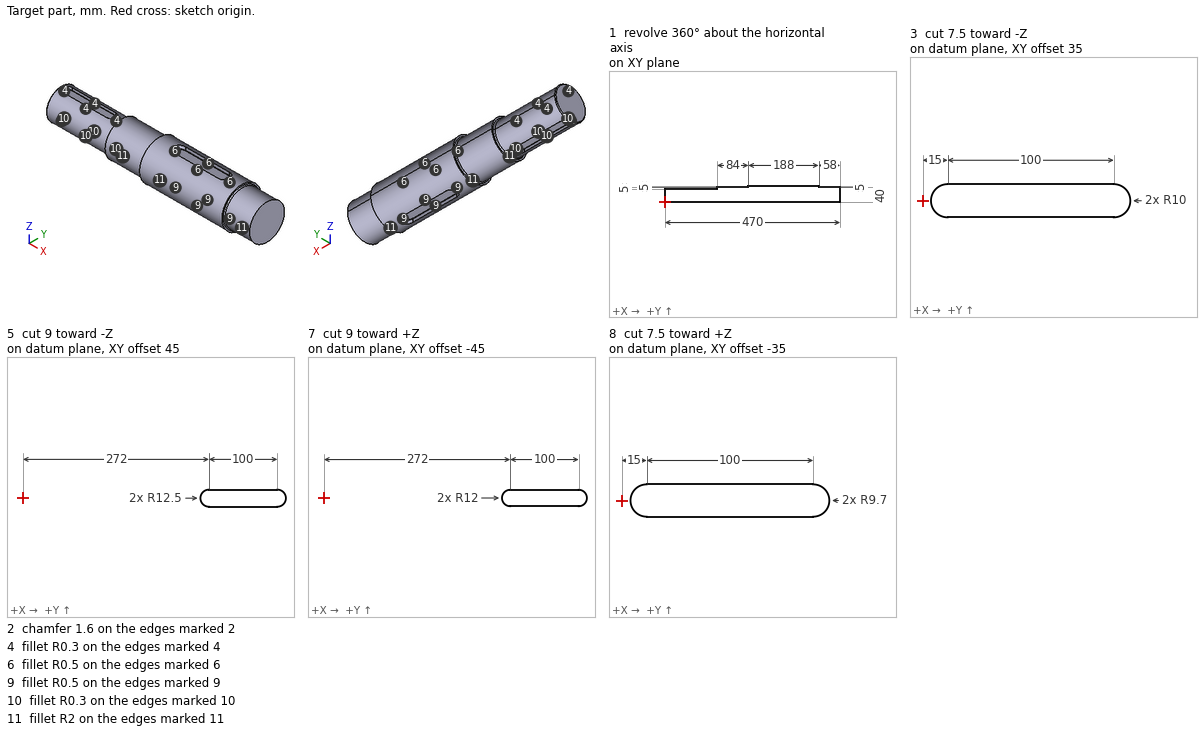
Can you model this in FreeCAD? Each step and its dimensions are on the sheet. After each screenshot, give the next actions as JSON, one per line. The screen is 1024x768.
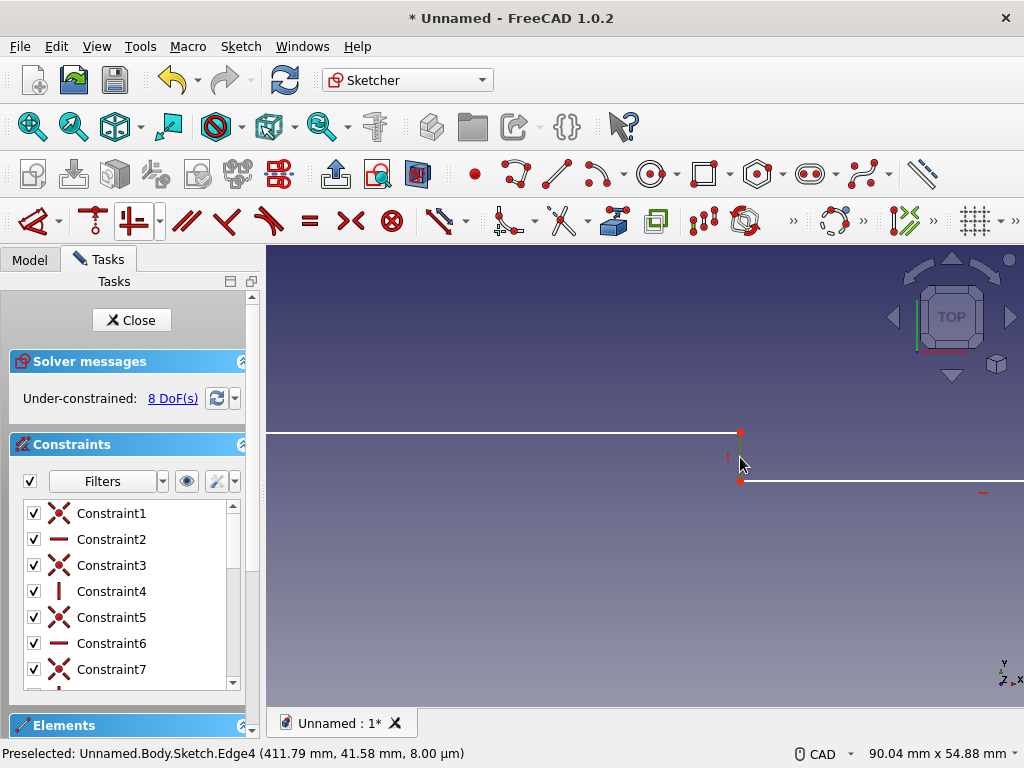
{"action": "key", "text": "i"}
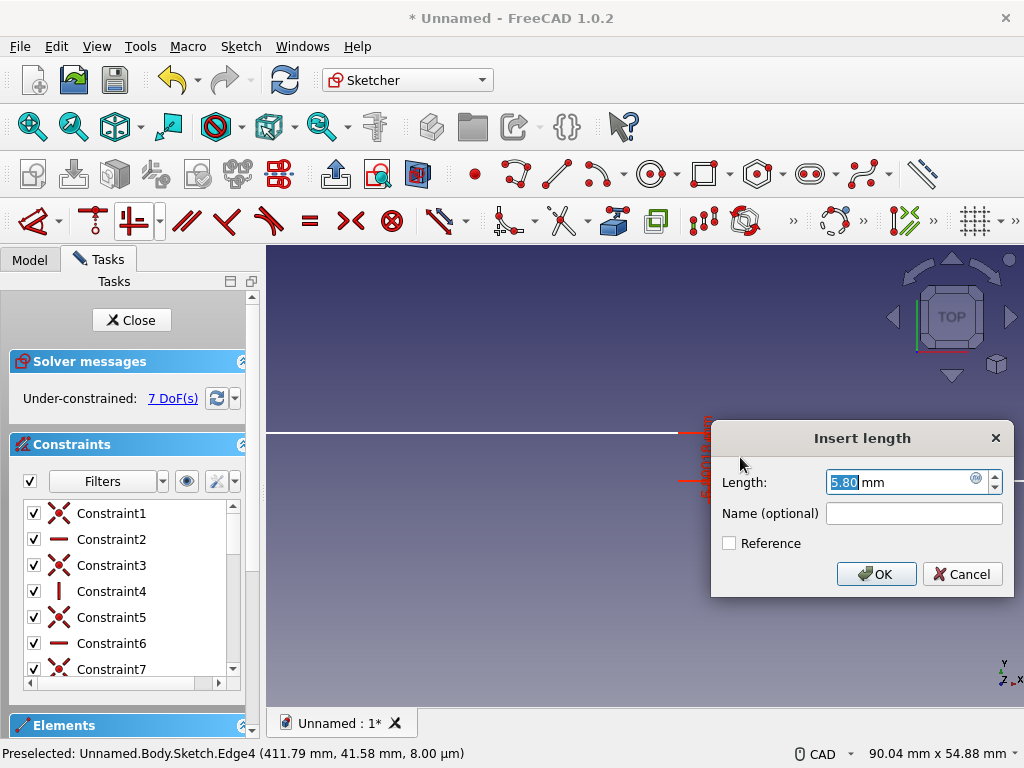
{"action": "type", "text": "5"}
{"action": "key", "text": "Return"}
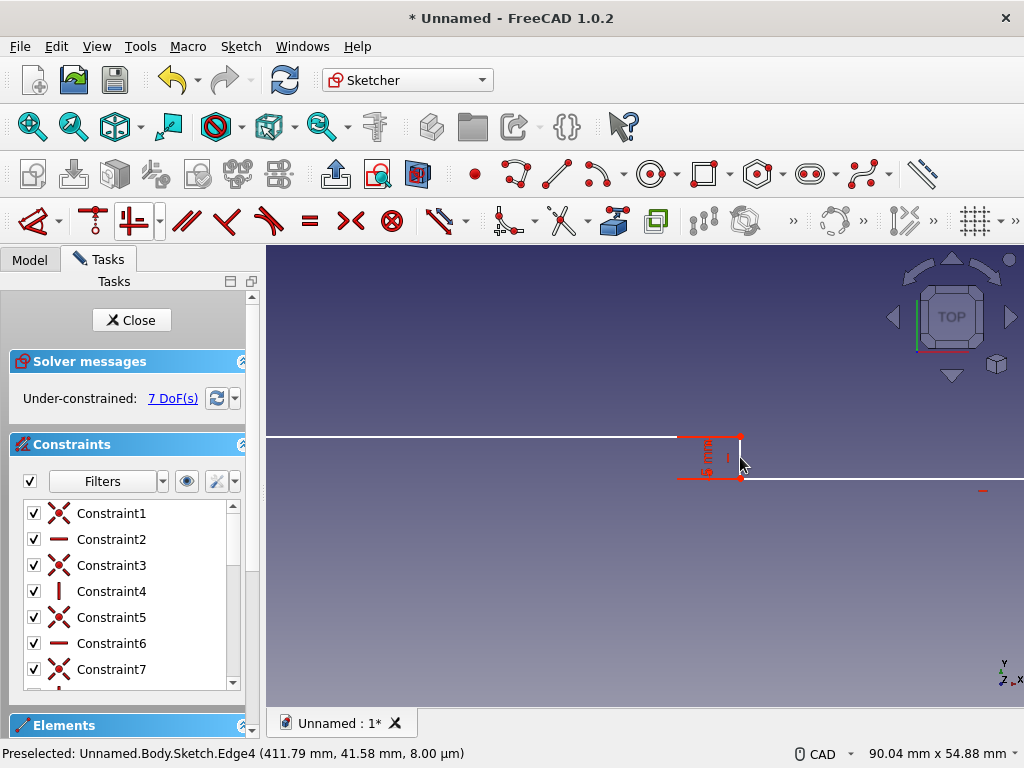
{"action": "scroll", "coordinate": [742, 458], "scroll_direction": "down", "scroll_amount": 11}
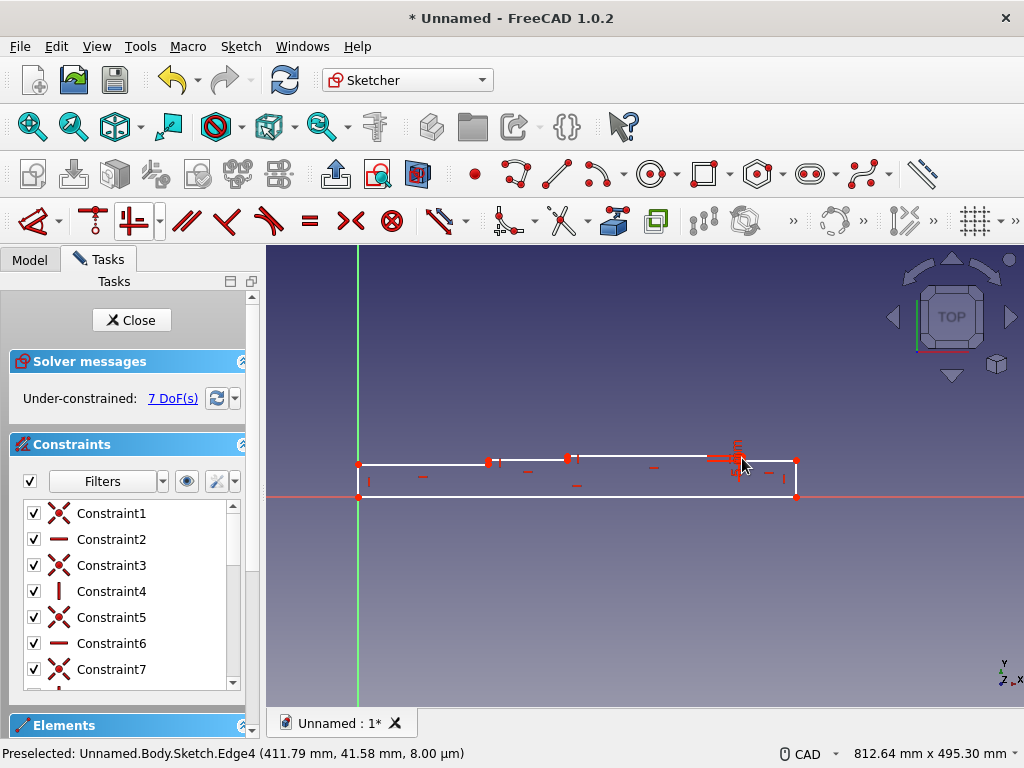
{"action": "scroll", "coordinate": [567, 457], "scroll_direction": "up", "scroll_amount": 13}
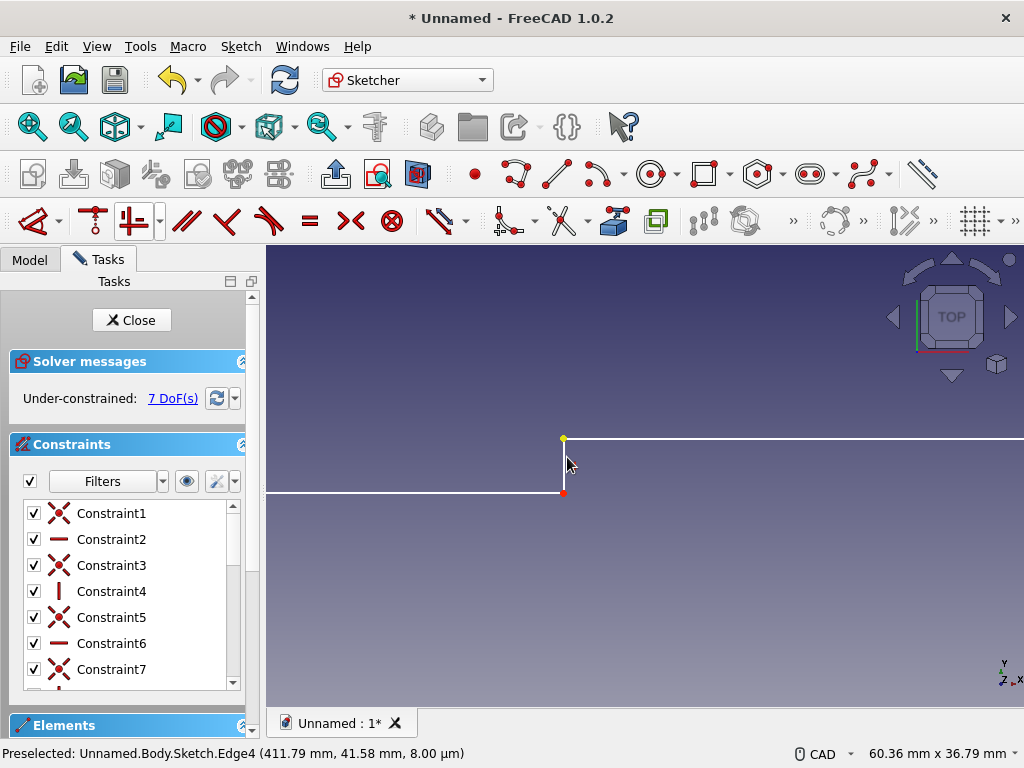
{"action": "left_click", "coordinate": [564, 455]}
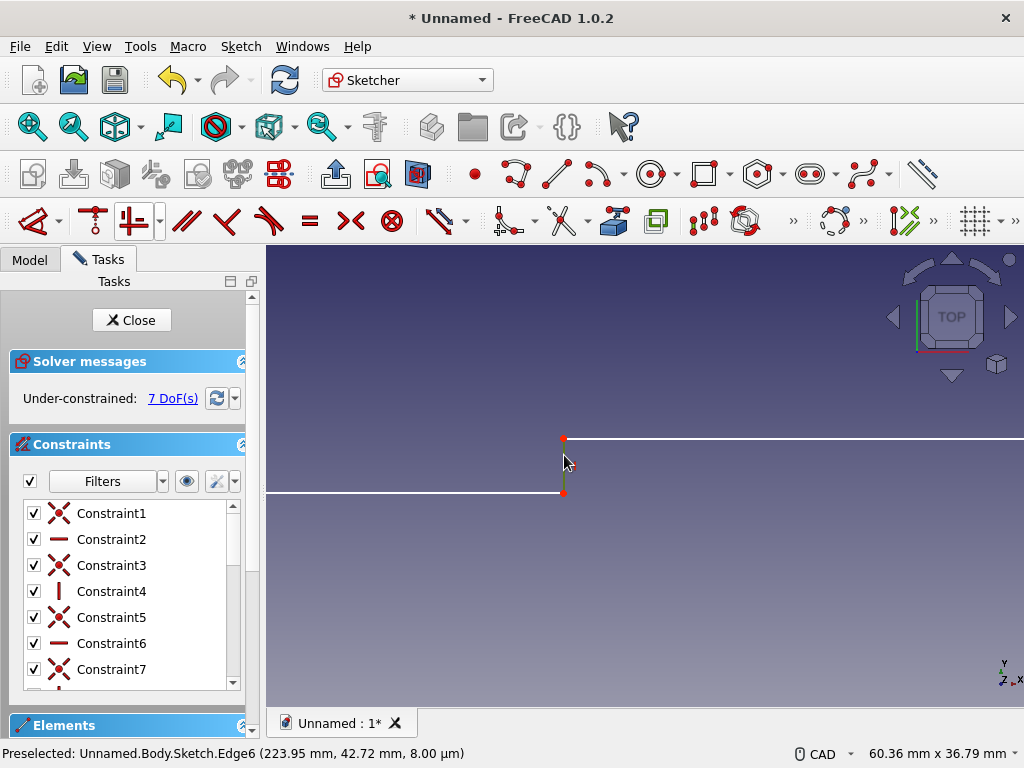
{"action": "key", "text": "i"}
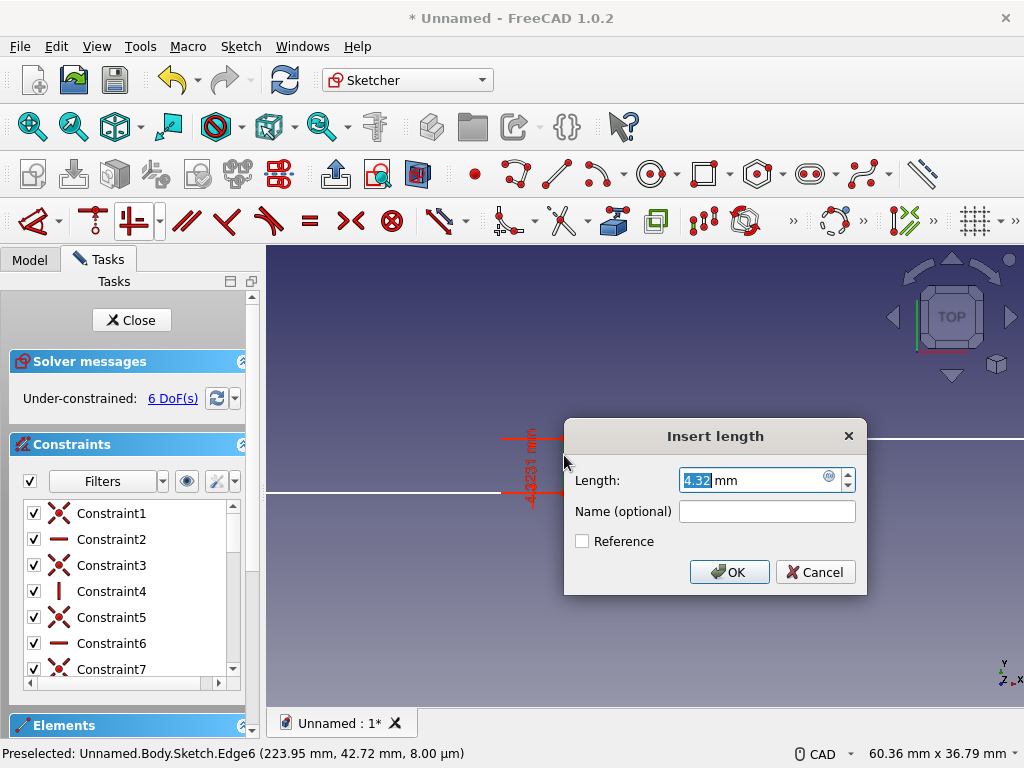
{"action": "type", "text": "5"}
{"action": "key", "text": "Return"}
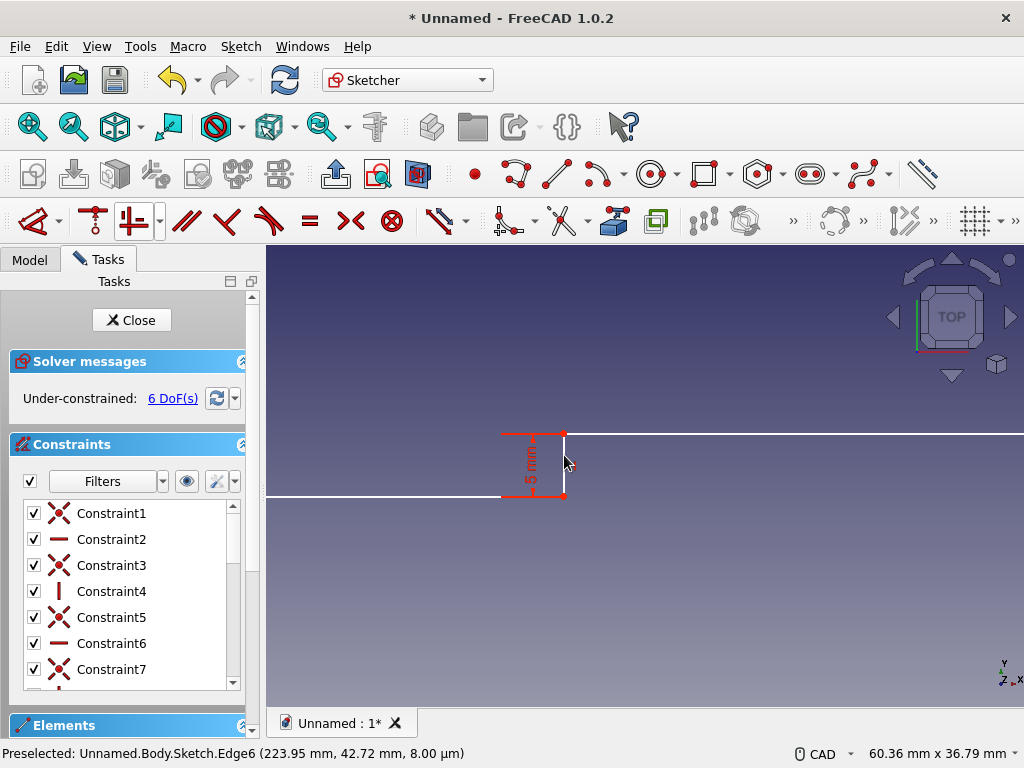
{"action": "scroll", "coordinate": [566, 457], "scroll_direction": "down", "scroll_amount": 13}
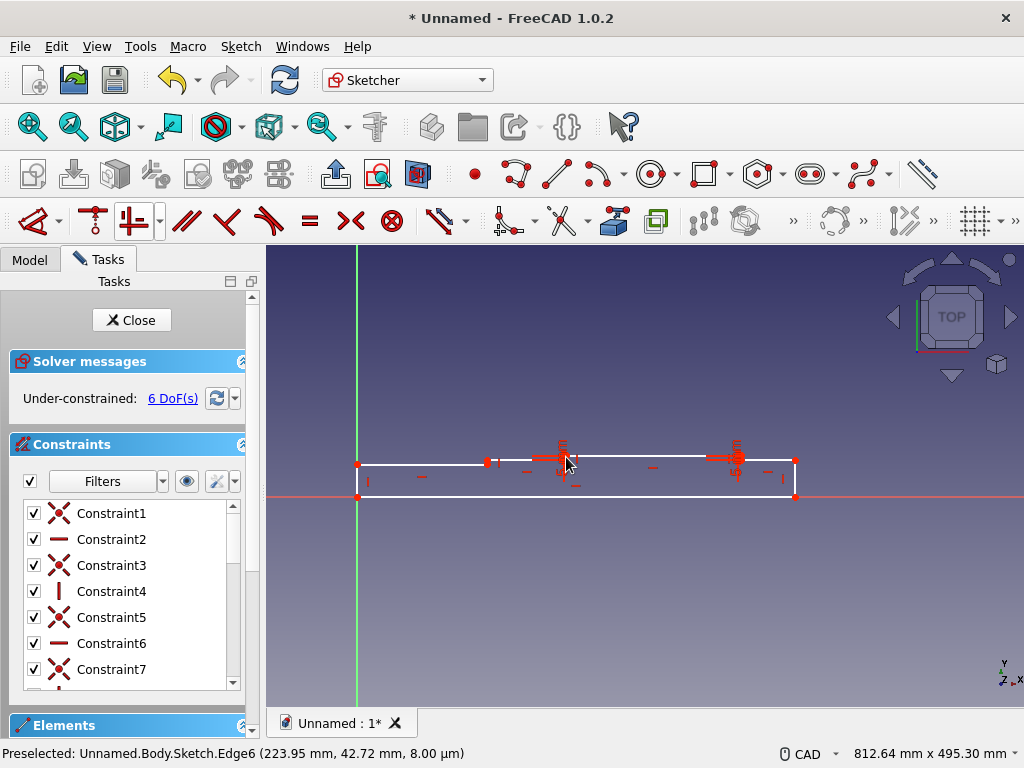
{"action": "scroll", "coordinate": [488, 462], "scroll_direction": "up", "scroll_amount": 12}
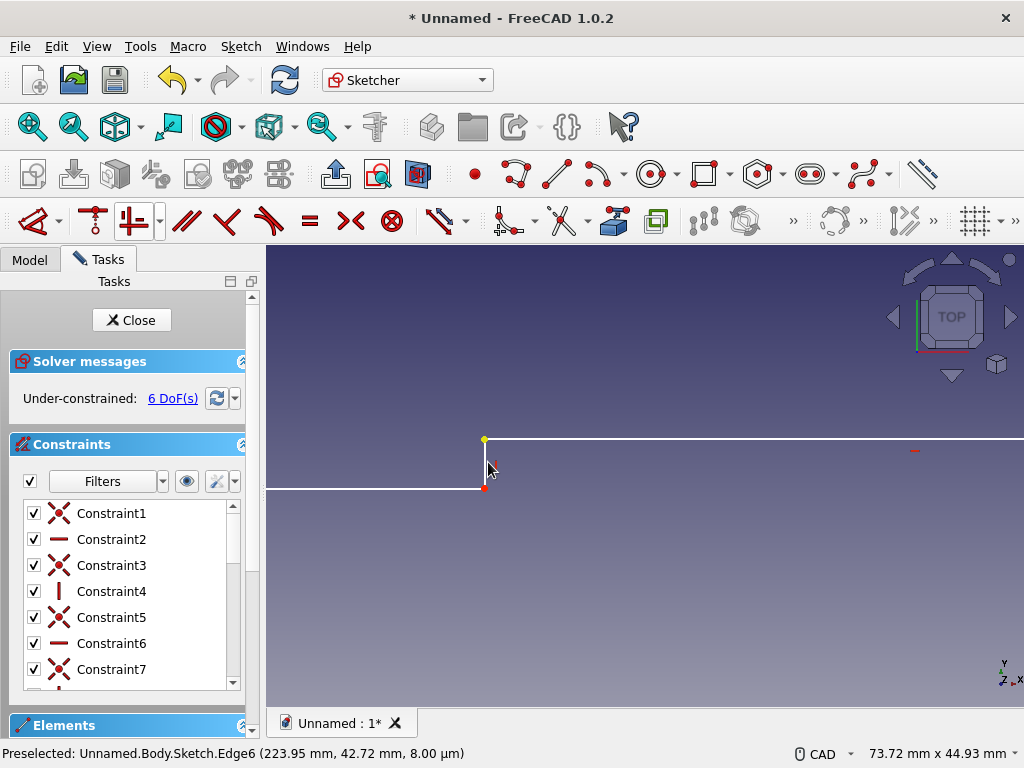
{"action": "left_click", "coordinate": [485, 454]}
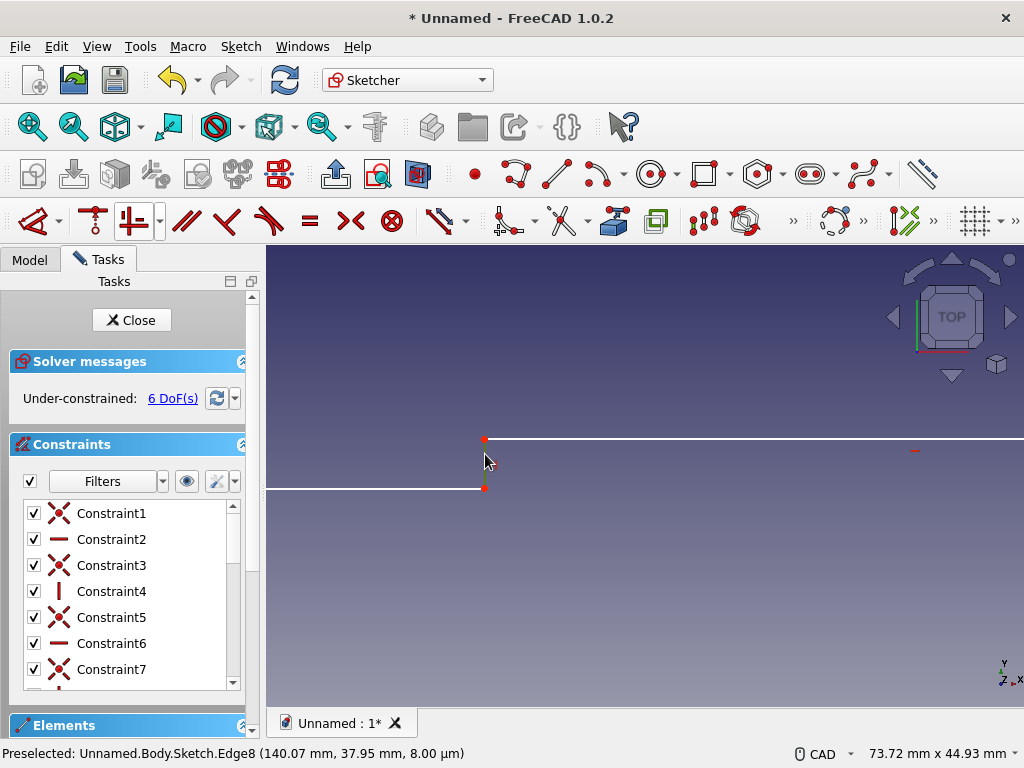
{"action": "left_click", "coordinate": [58, 222]}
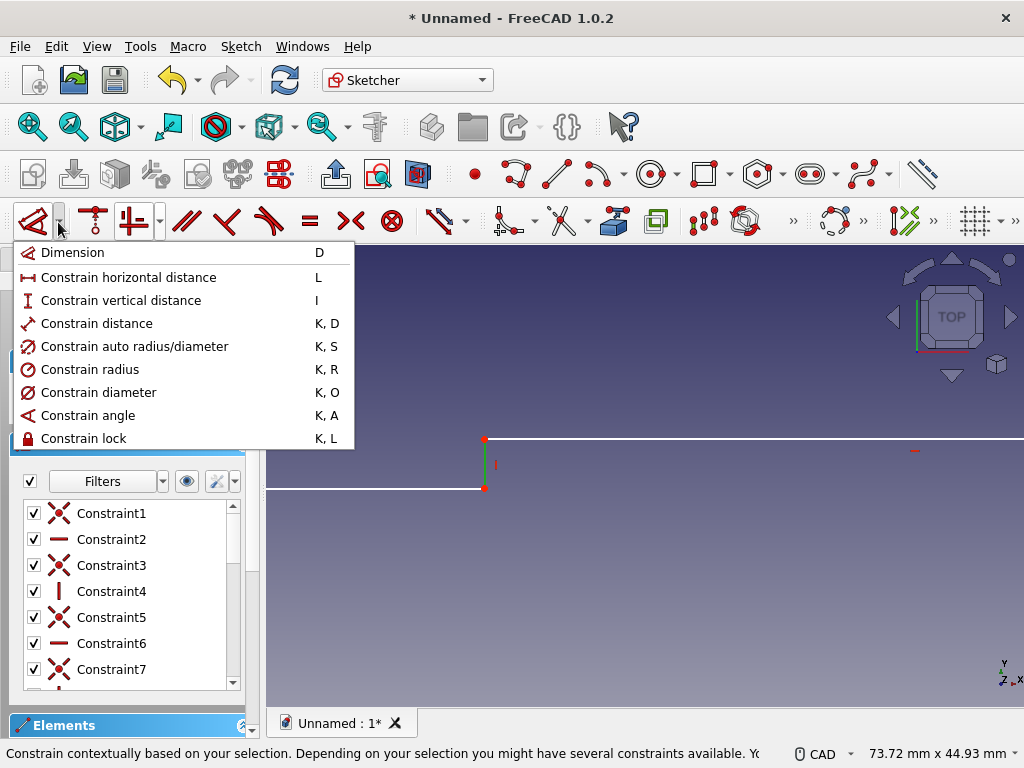
{"action": "left_click", "coordinate": [184, 300]}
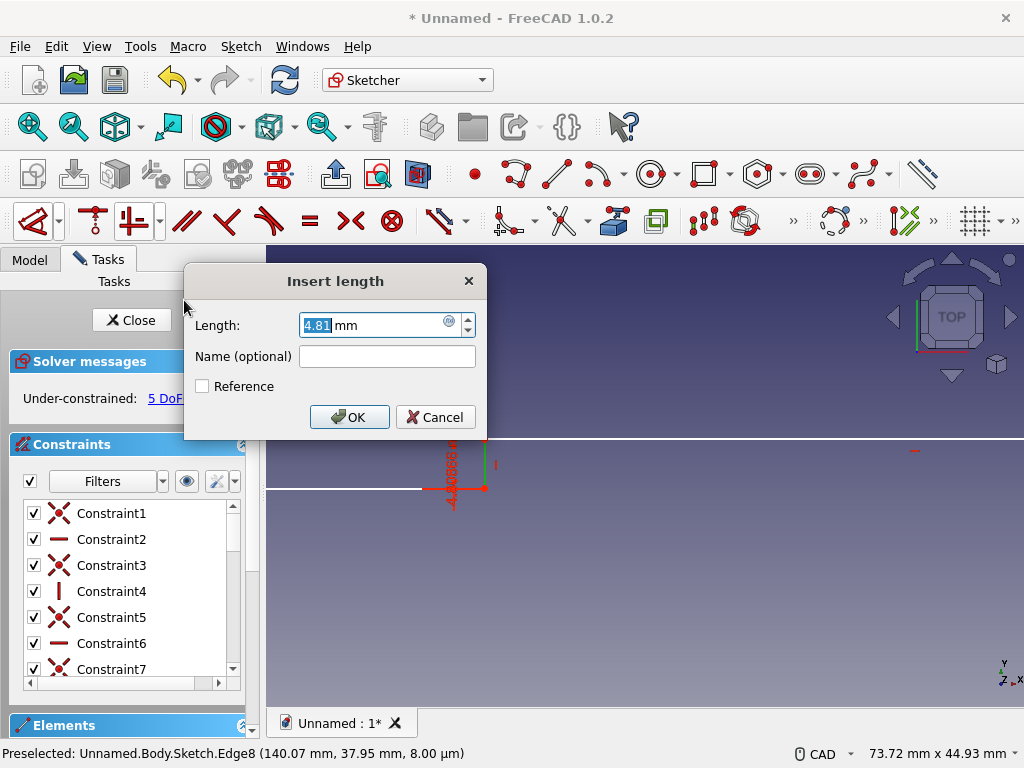
{"action": "type", "text": "5"}
{"action": "key", "text": "Return"}